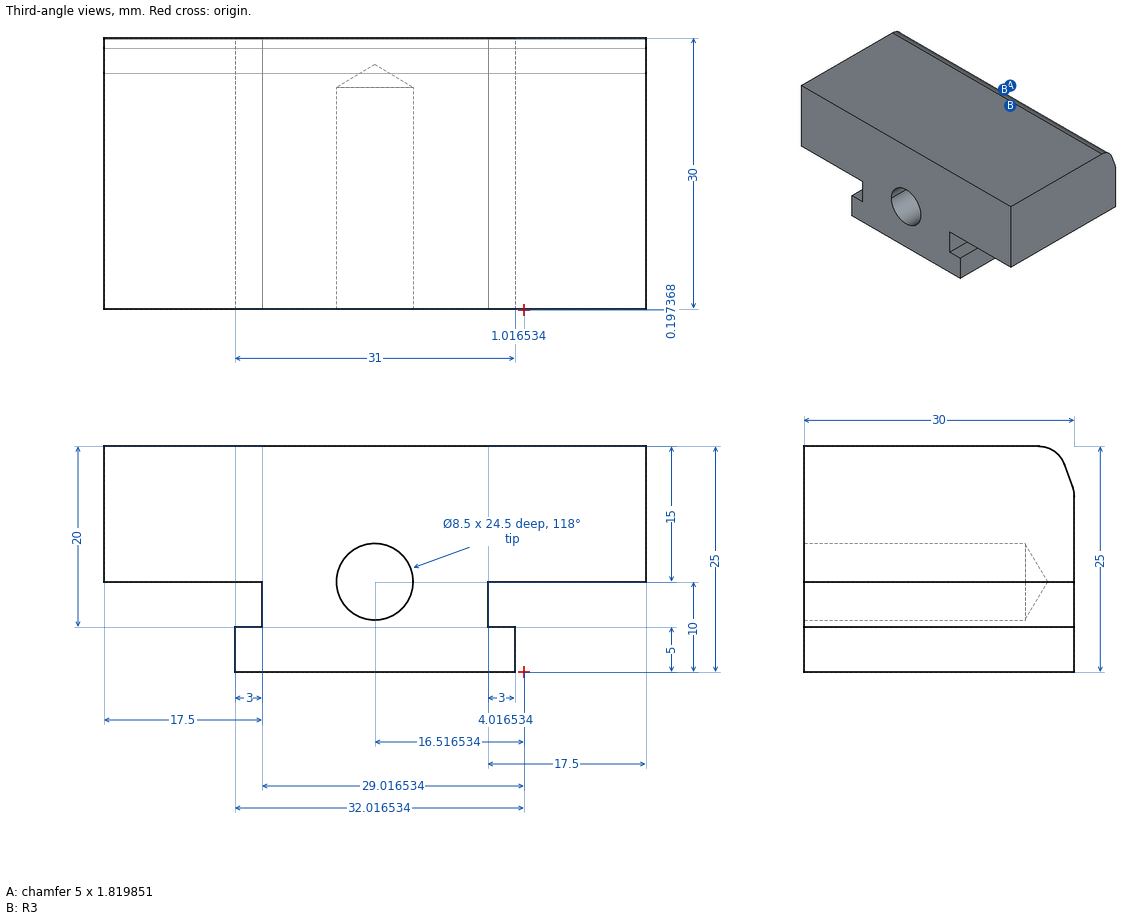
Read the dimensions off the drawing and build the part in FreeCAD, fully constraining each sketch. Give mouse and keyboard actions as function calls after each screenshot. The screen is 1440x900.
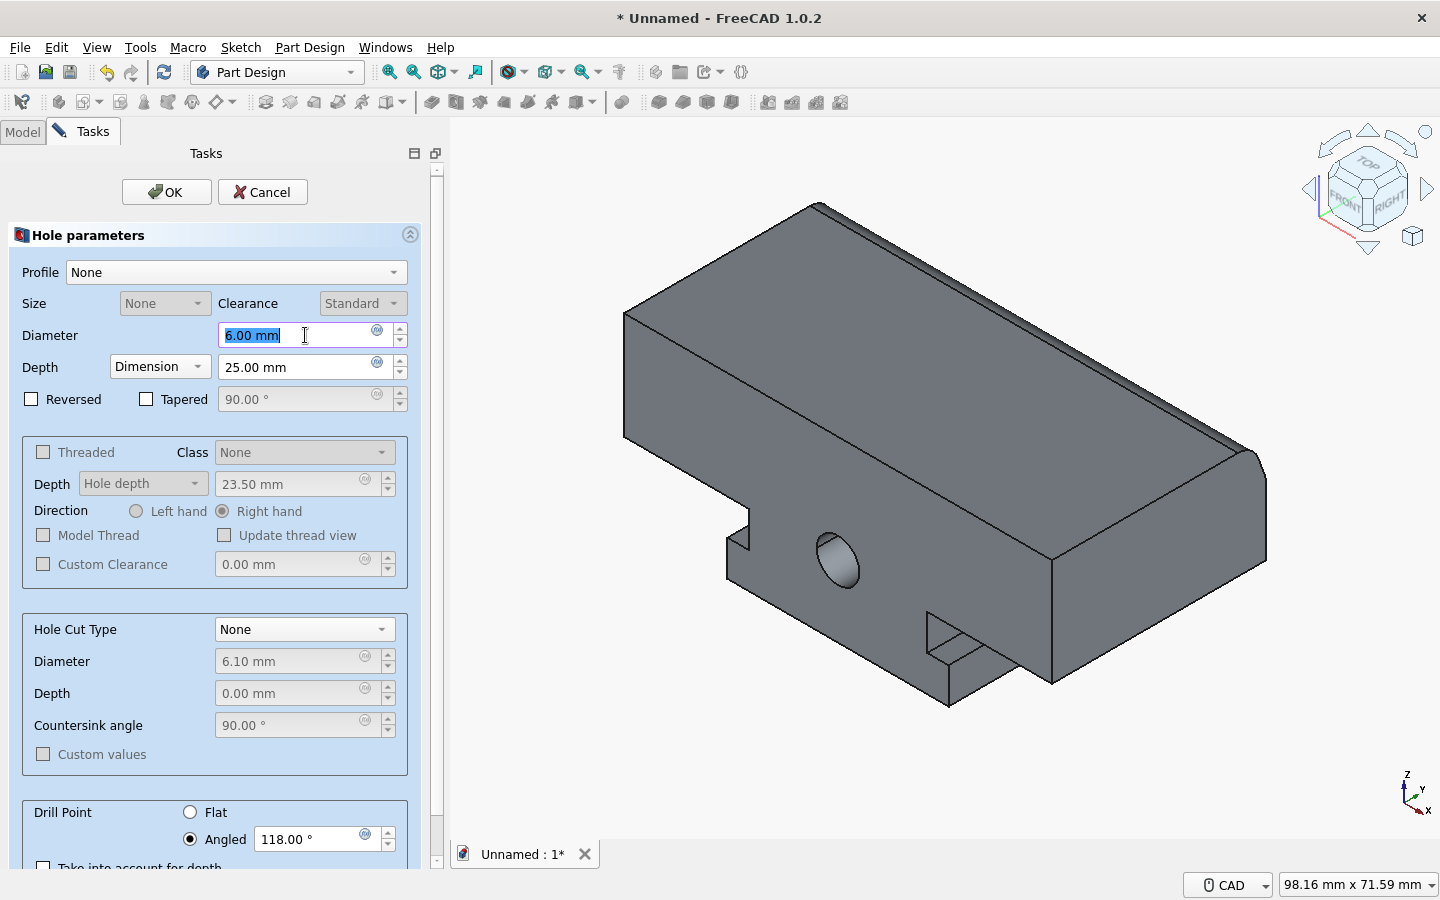
text(8.5)
key(Tab)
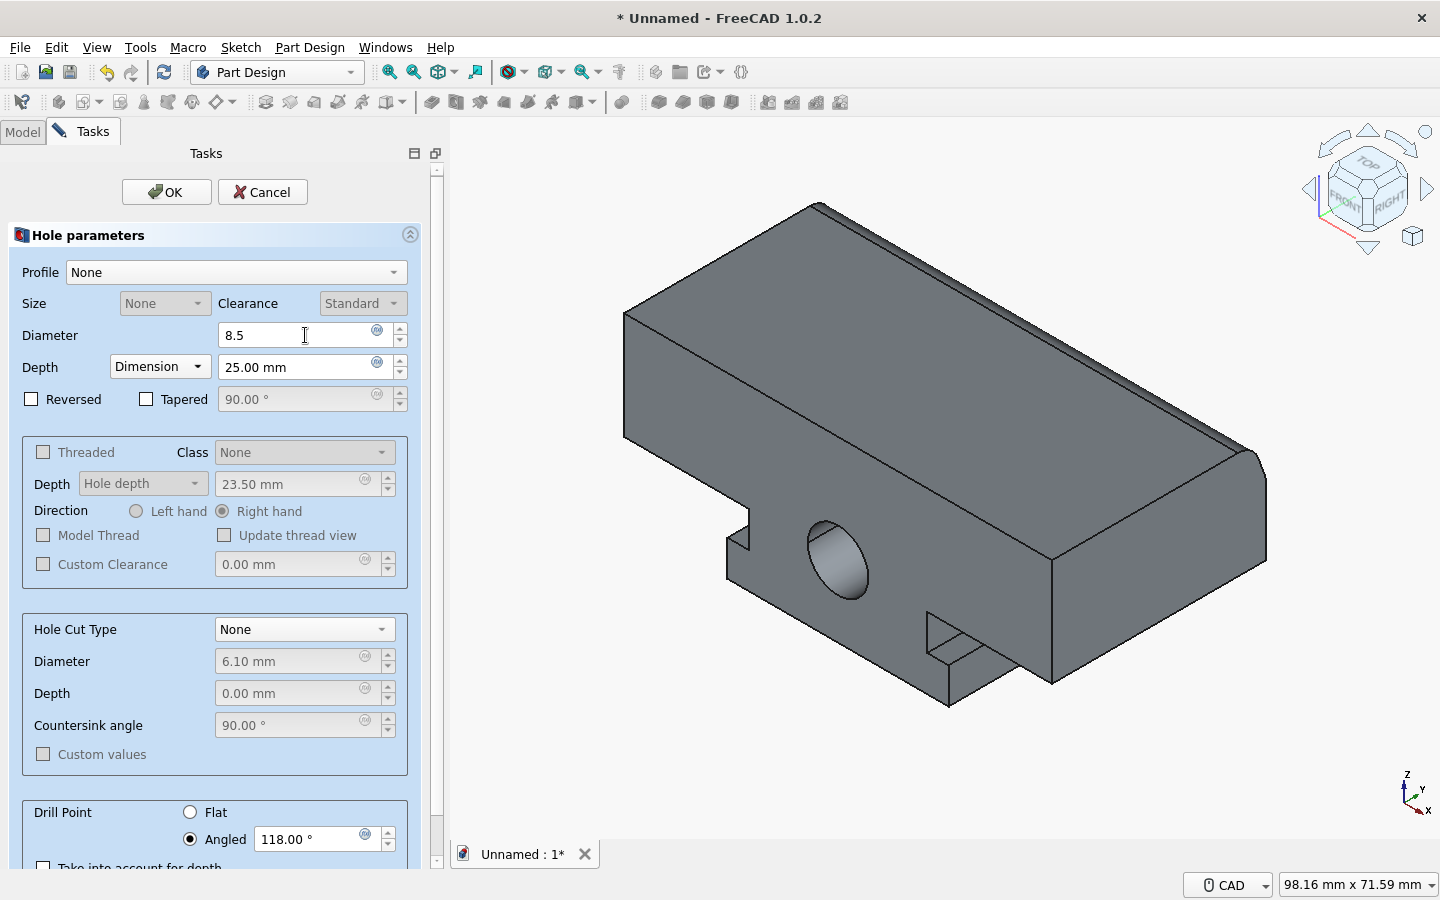
triple_click(305, 367)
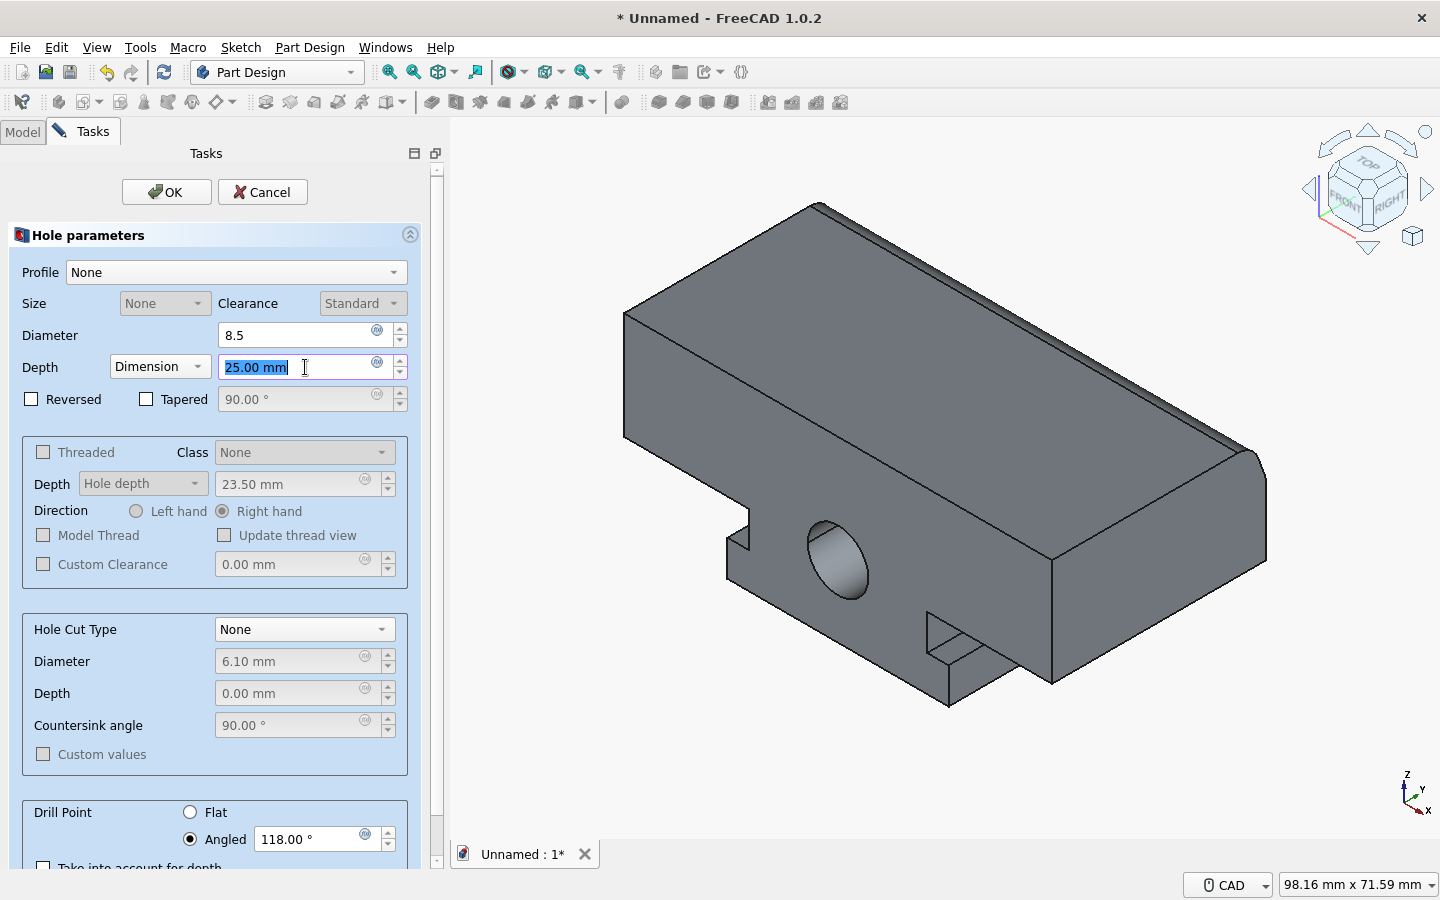
text(24.5)
key(Tab)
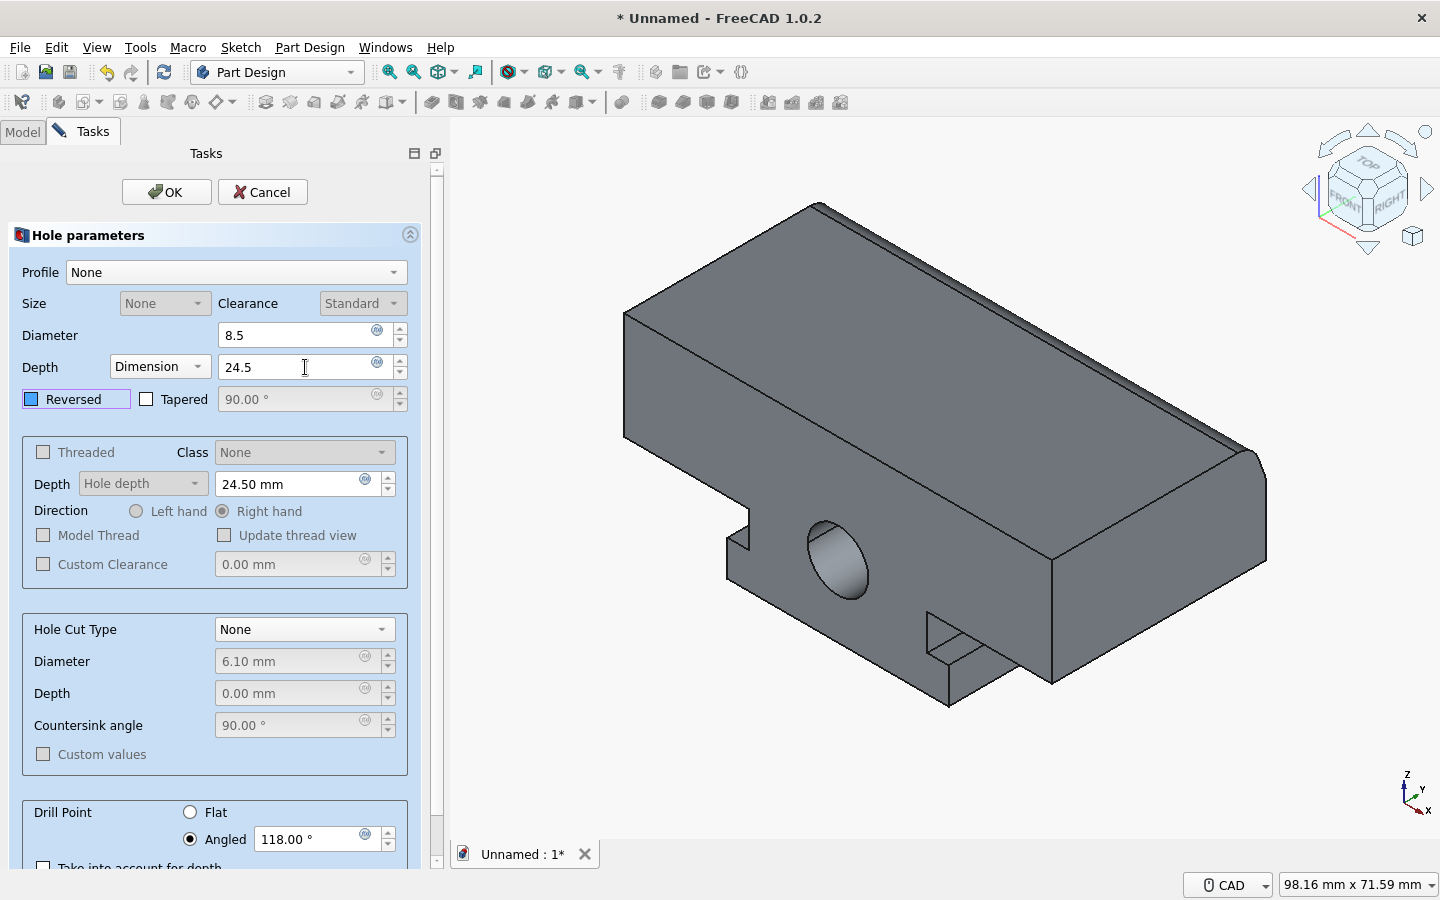
click(167, 192)